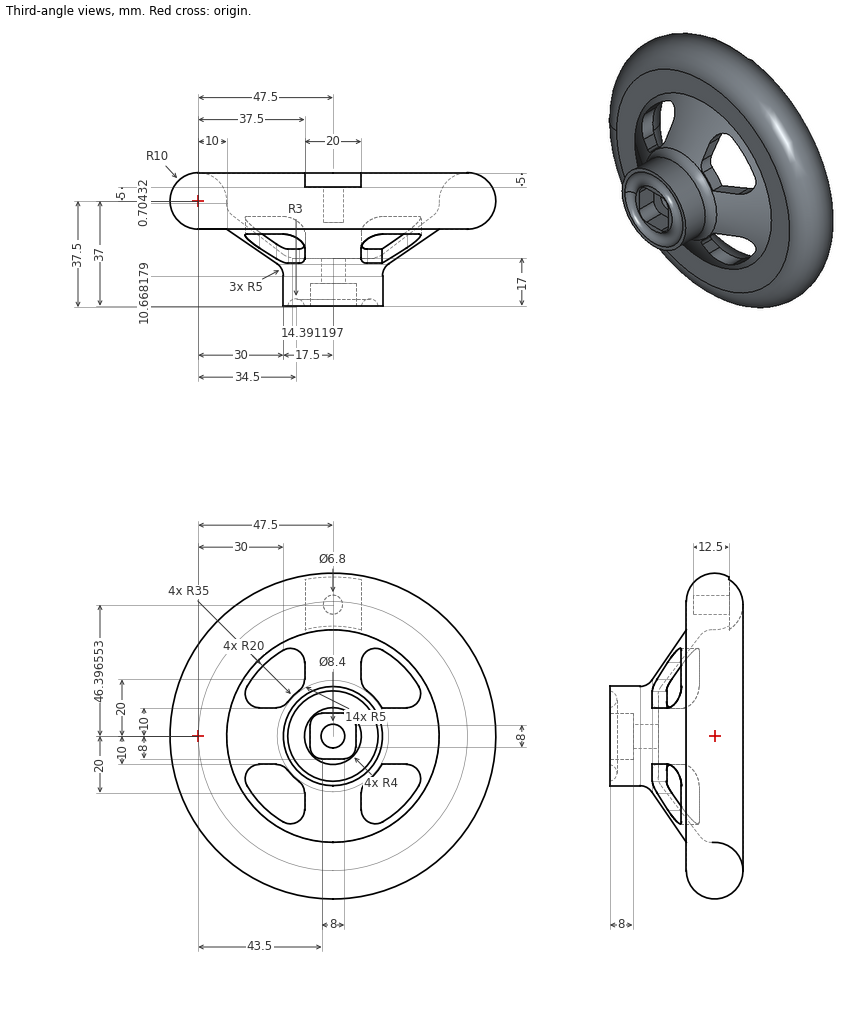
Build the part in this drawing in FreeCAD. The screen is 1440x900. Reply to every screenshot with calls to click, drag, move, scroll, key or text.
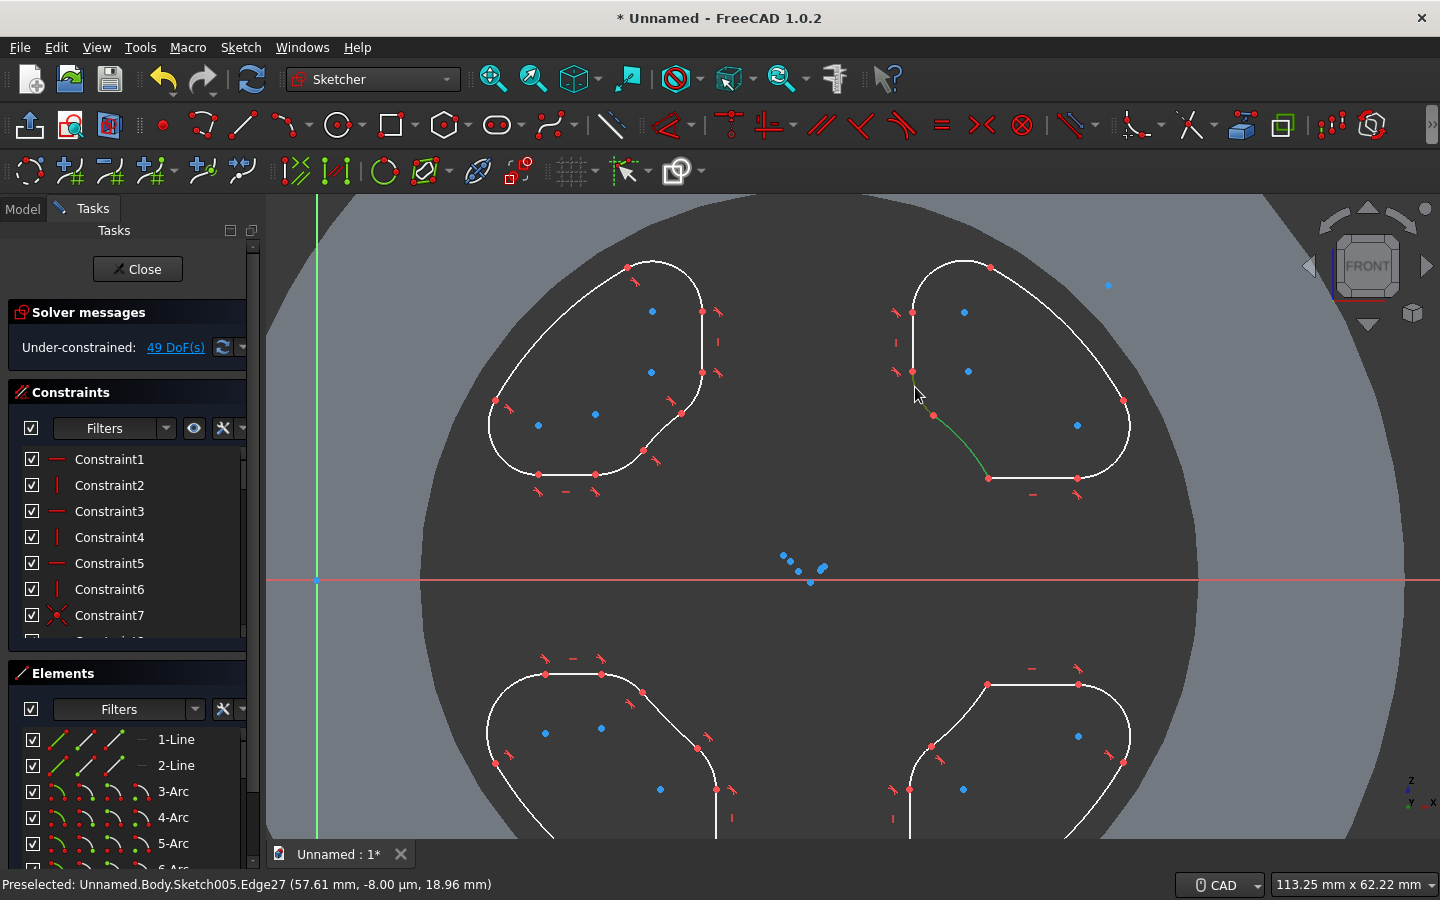
click(902, 126)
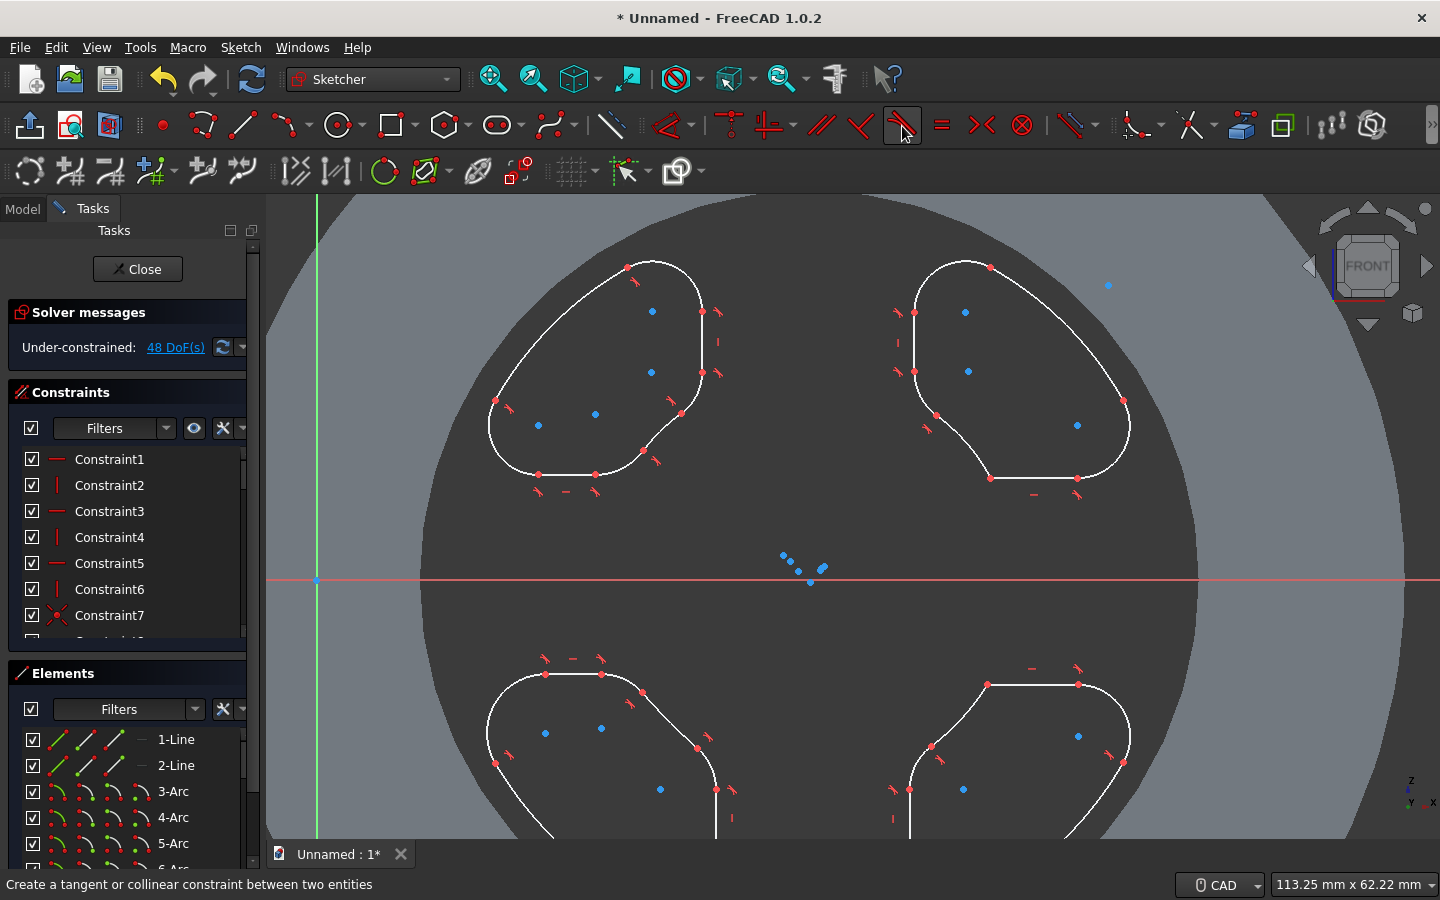
click(960, 262)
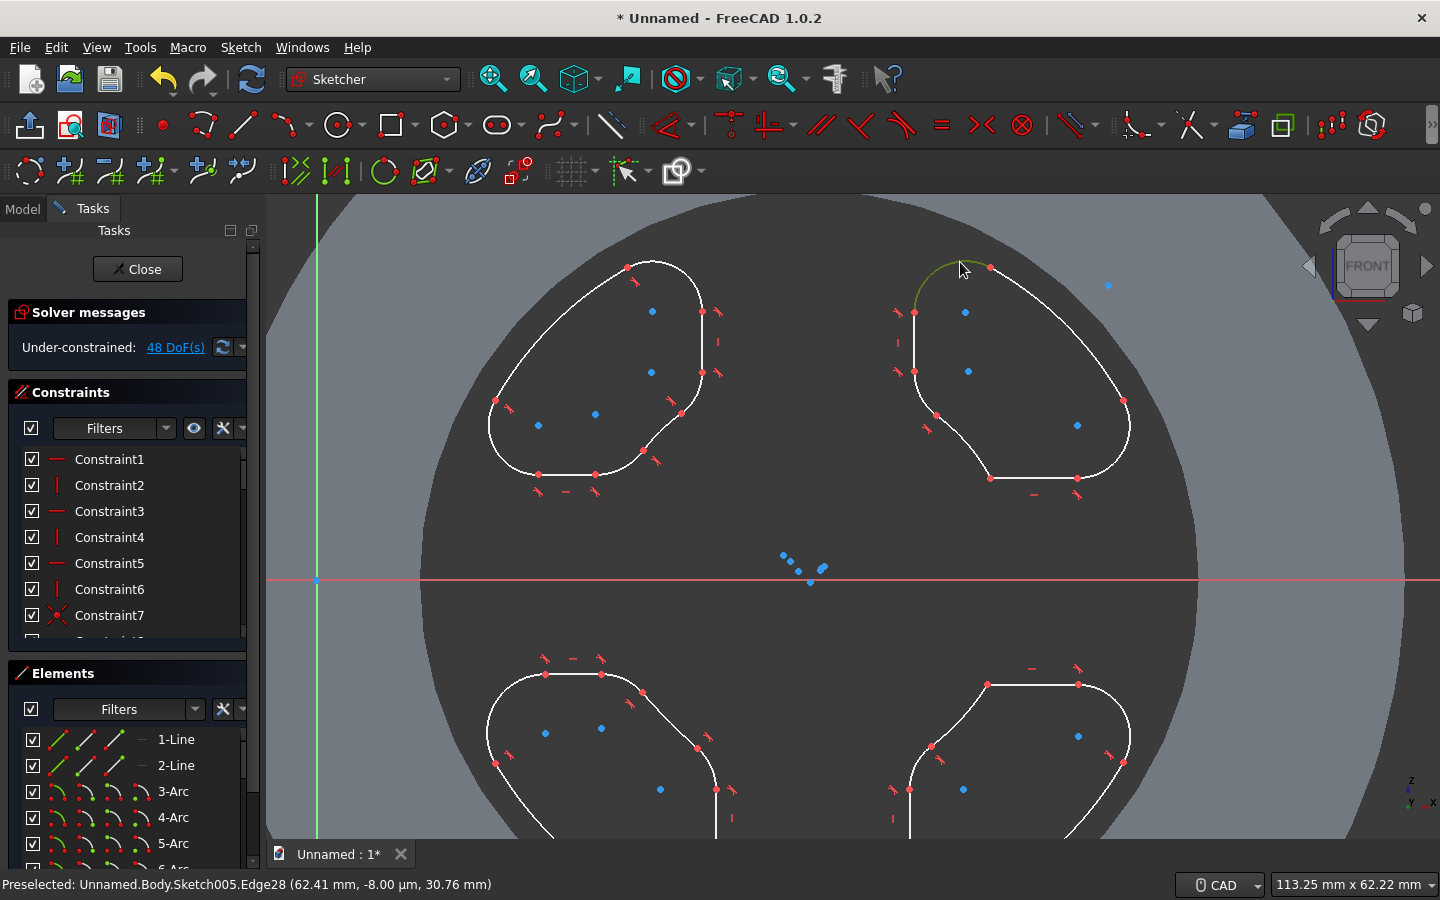
click(1091, 353)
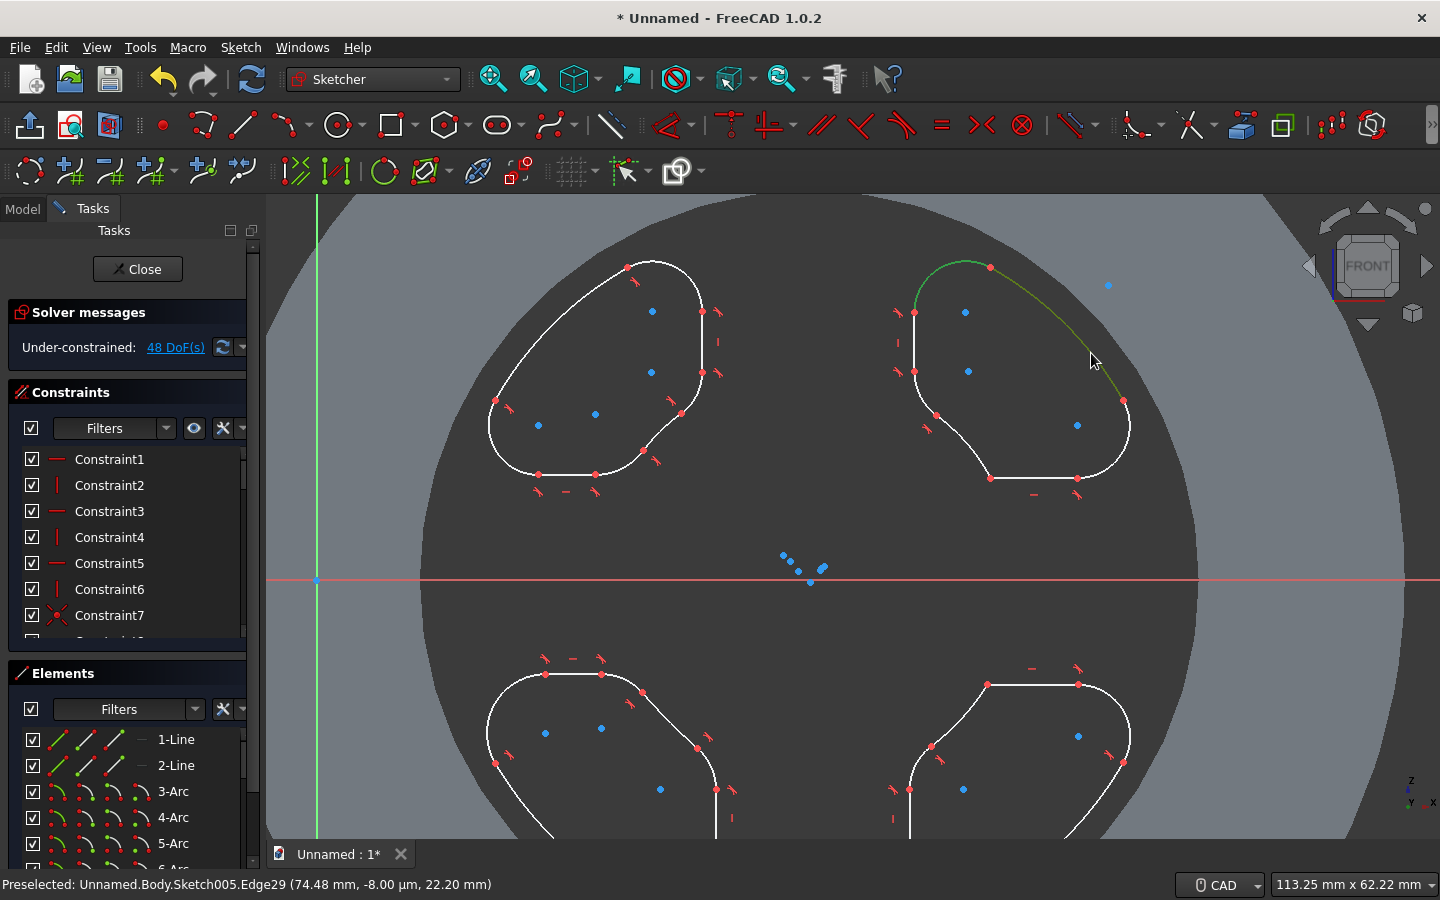
click(902, 126)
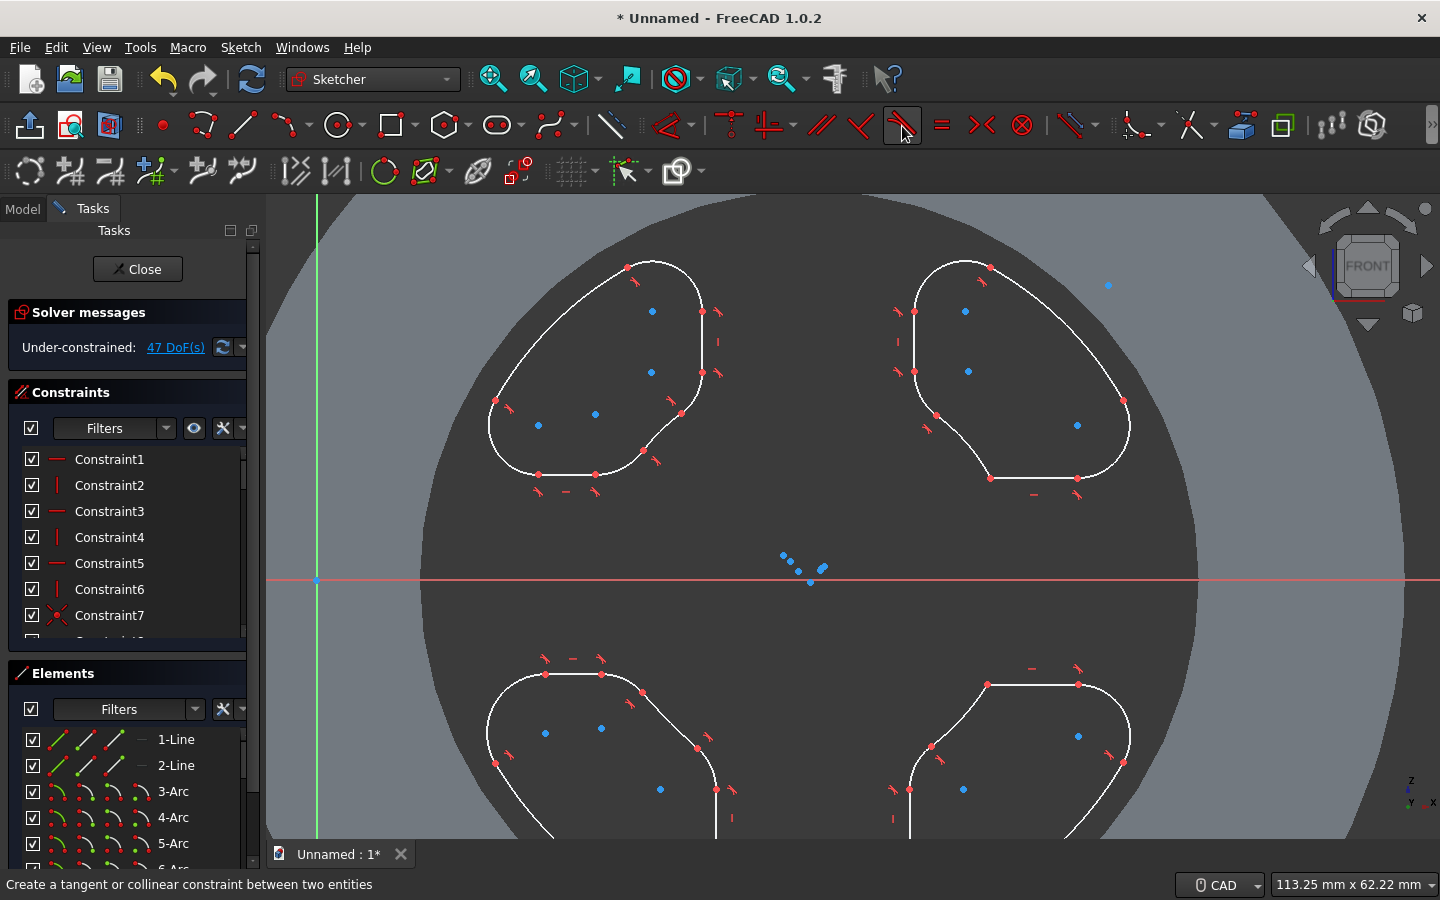
click(1091, 353)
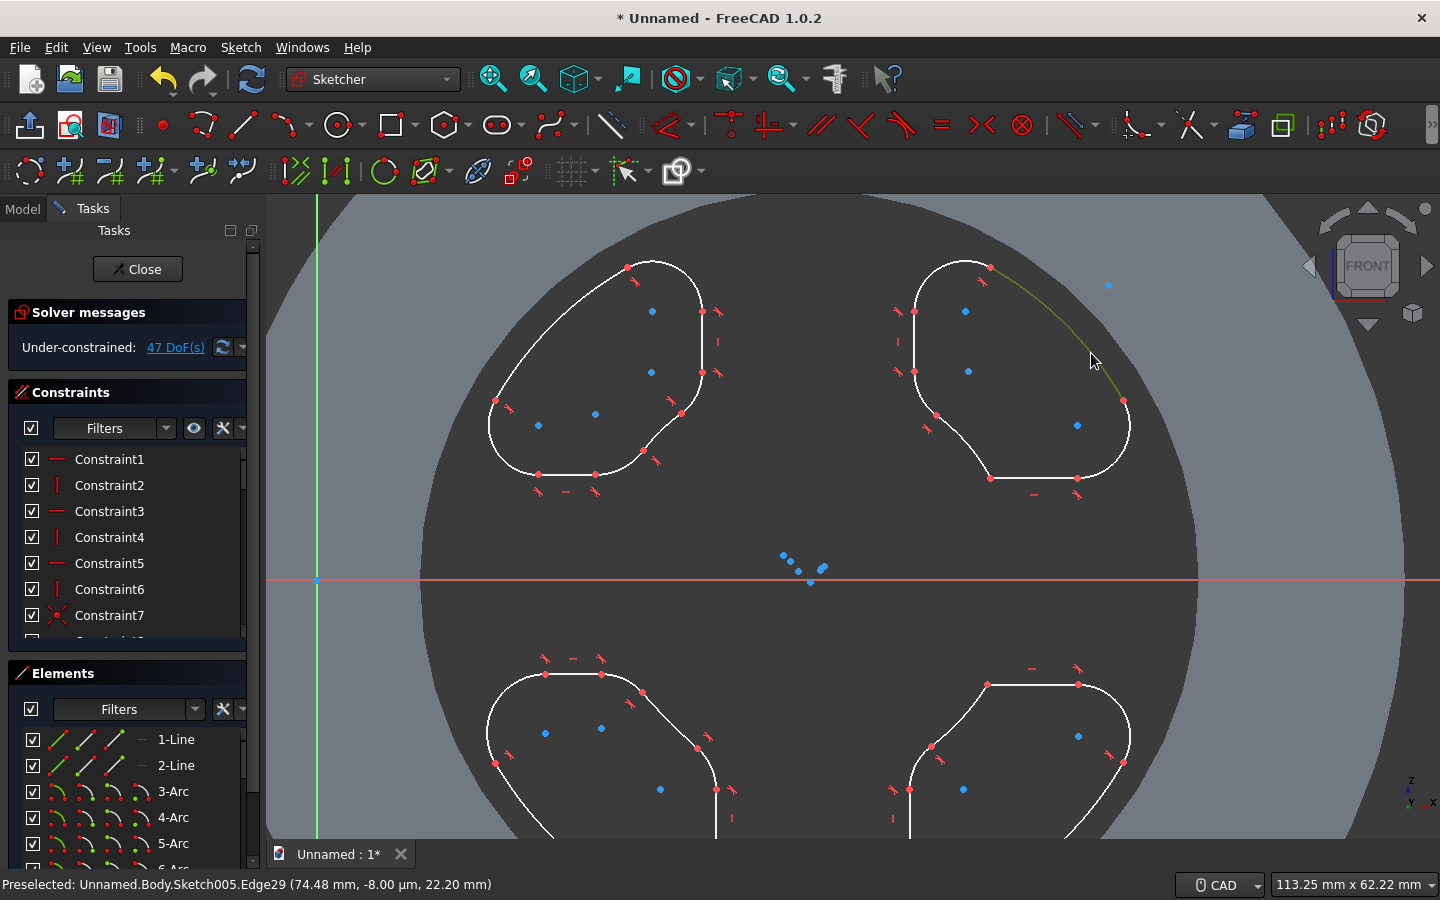
click(1108, 468)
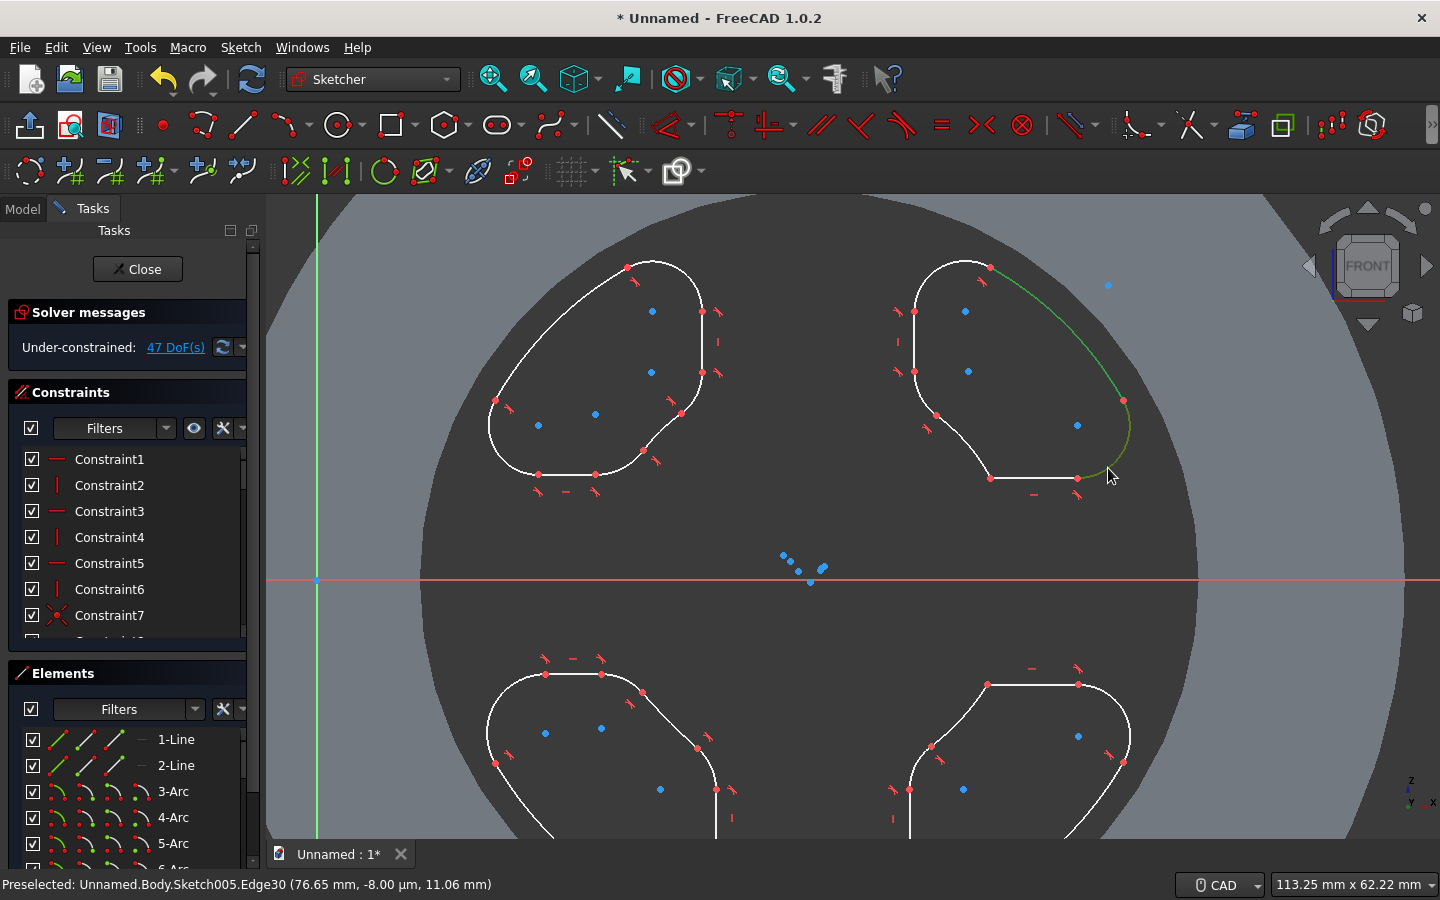
click(902, 126)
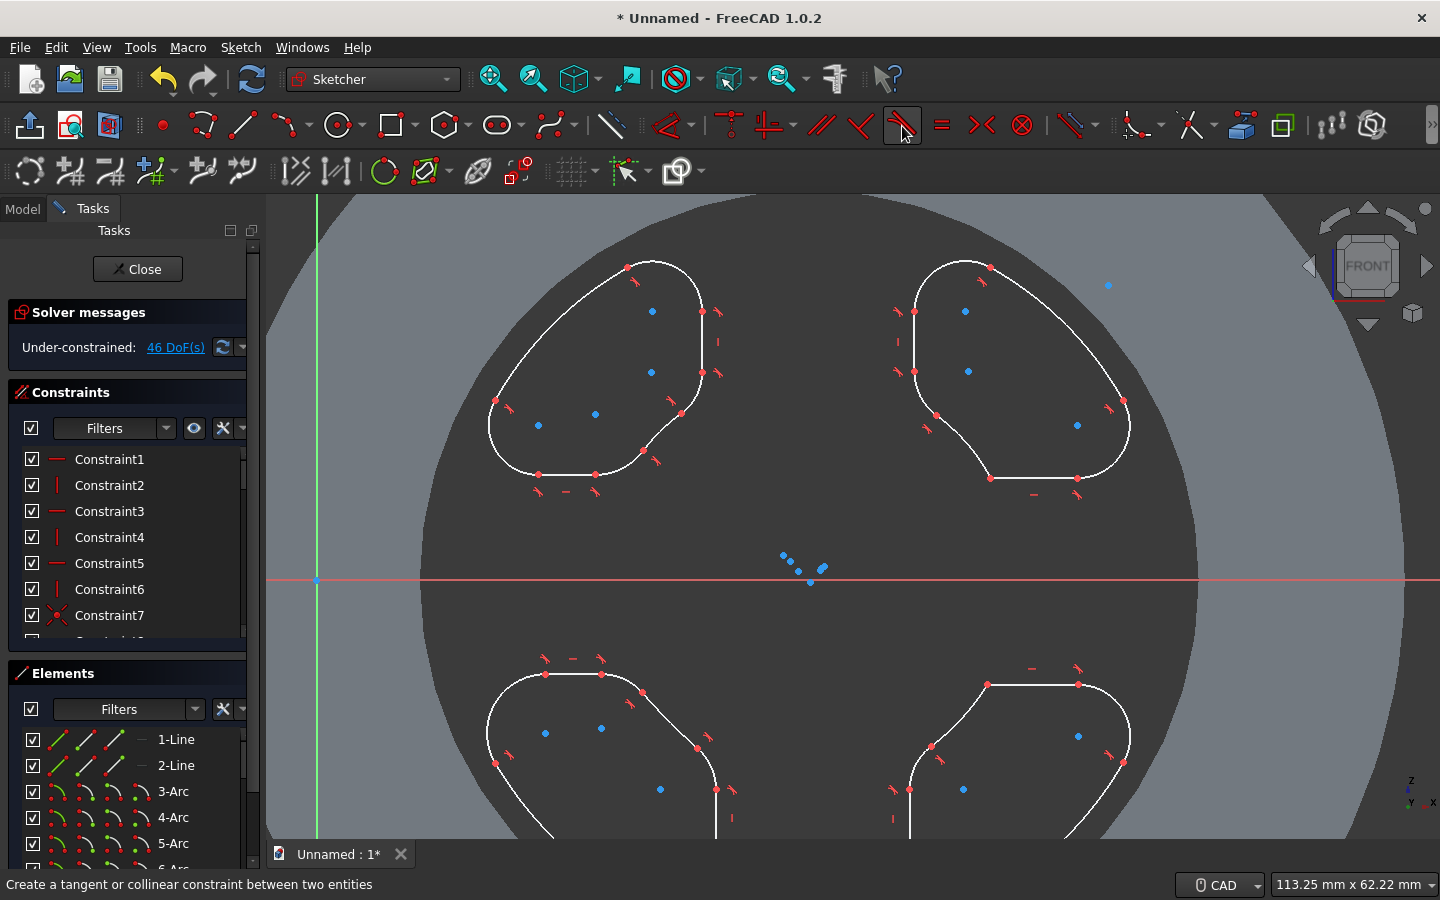
click(581, 300)